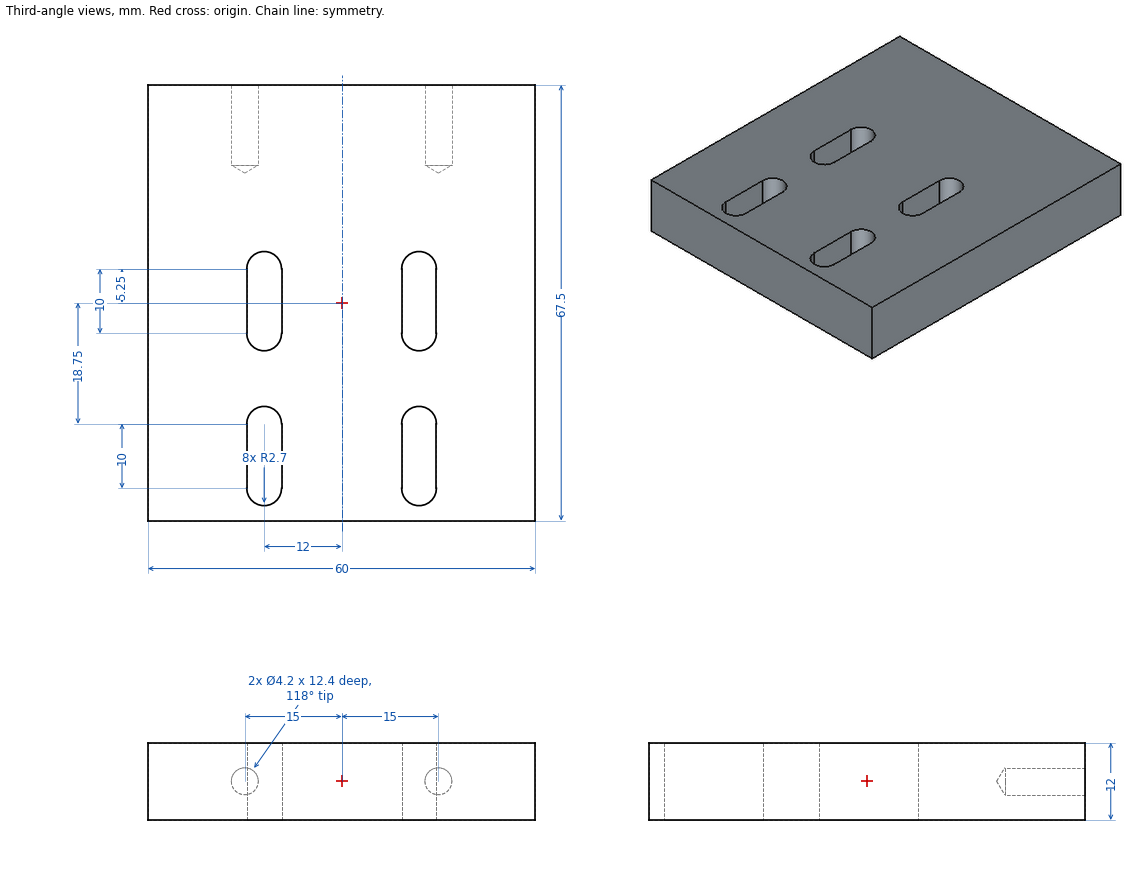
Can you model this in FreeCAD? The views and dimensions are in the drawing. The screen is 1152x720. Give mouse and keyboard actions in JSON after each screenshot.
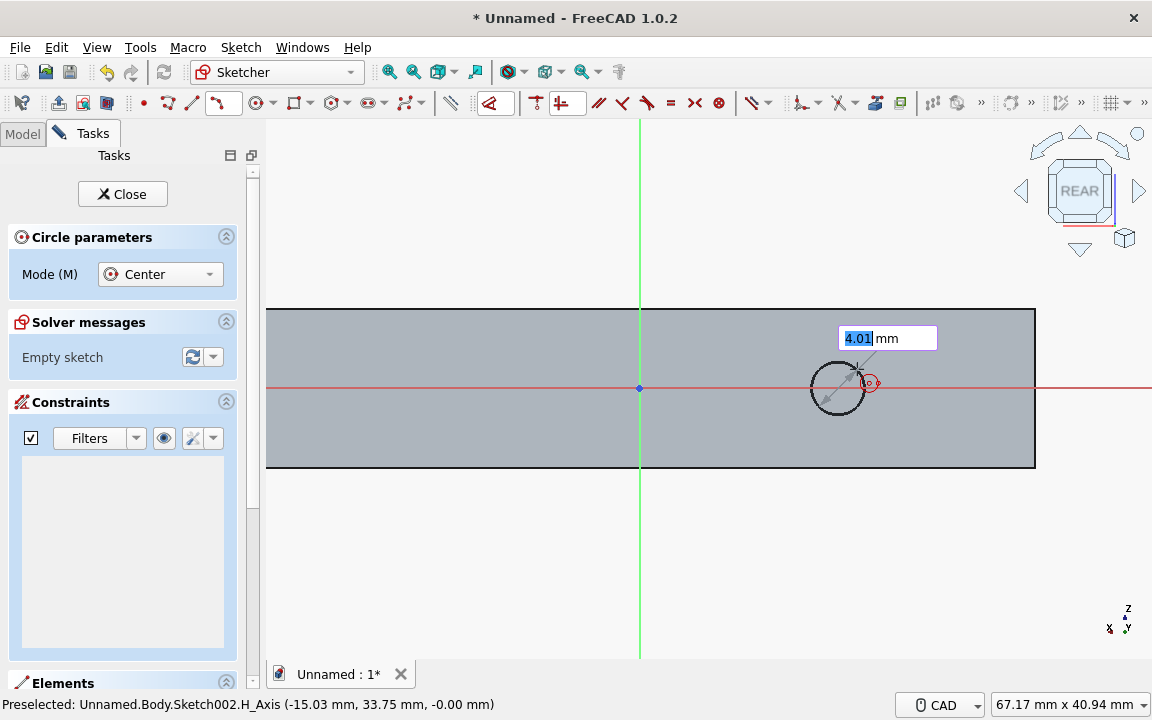
{"action": "type", "text": "4.2"}
{"action": "key", "text": "Return"}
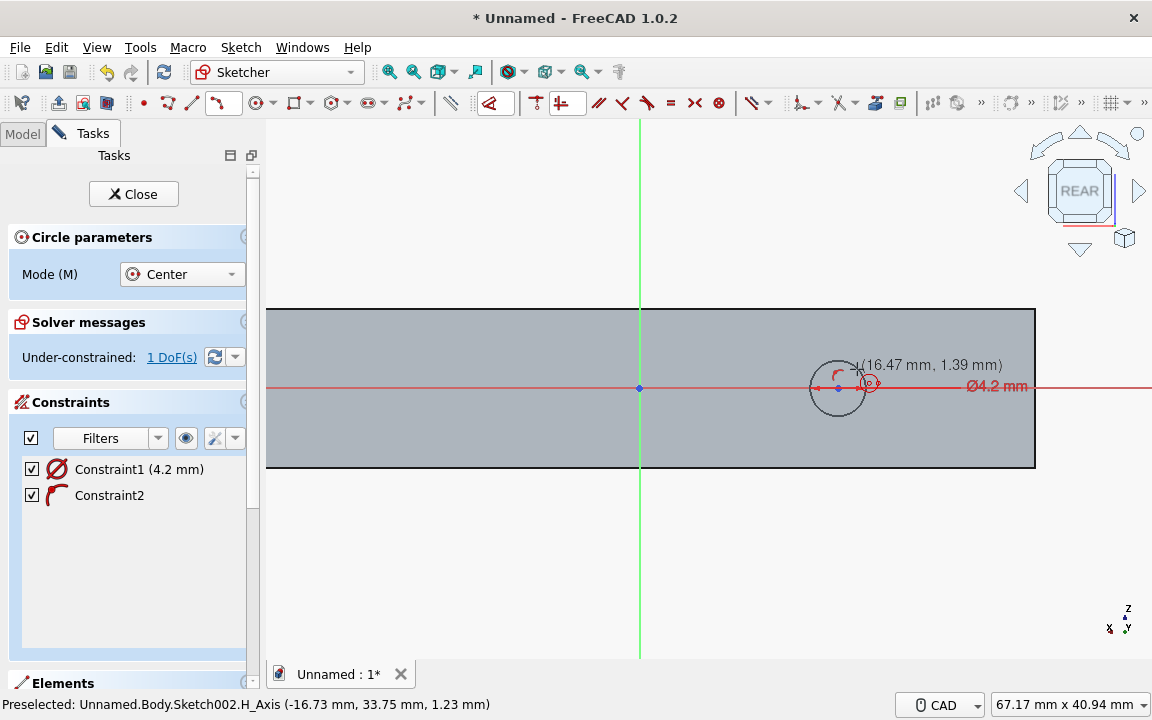
{"action": "left_click", "coordinate": [442, 388]}
{"action": "mouse_move", "coordinate": [461, 369]}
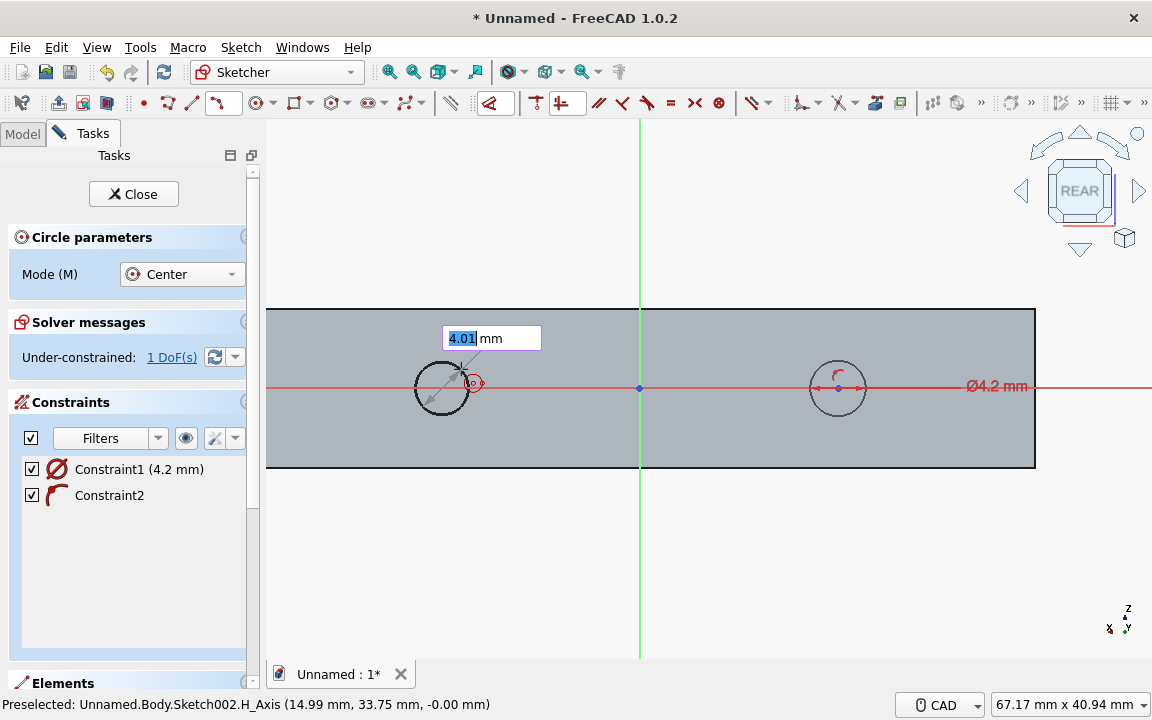
{"action": "type", "text": "4.2"}
{"action": "key", "text": "Return"}
{"action": "key", "text": "Escape"}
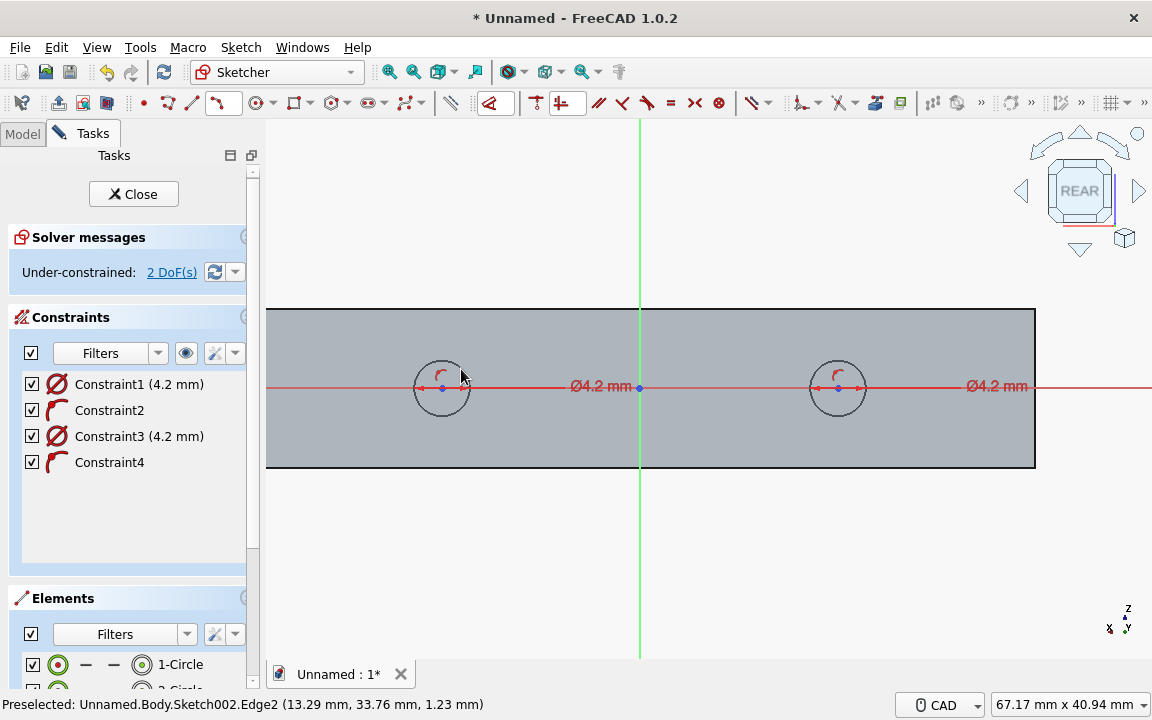
{"action": "left_click", "coordinate": [838, 388]}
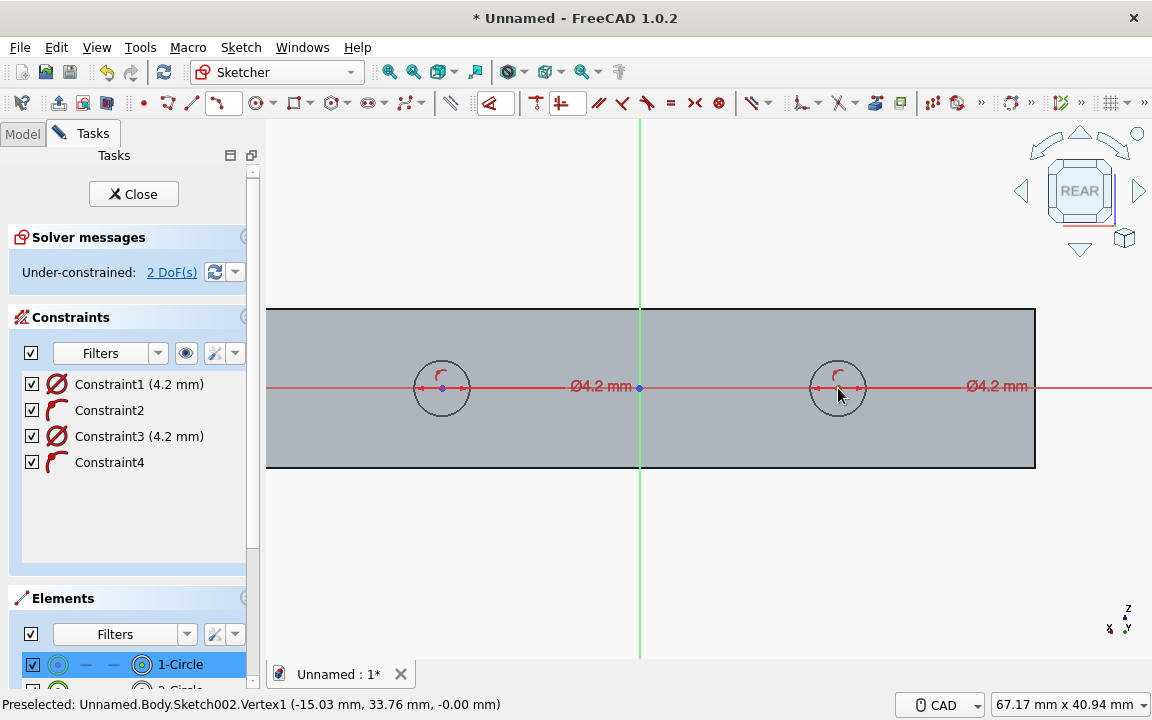
{"action": "left_click", "coordinate": [508, 104]}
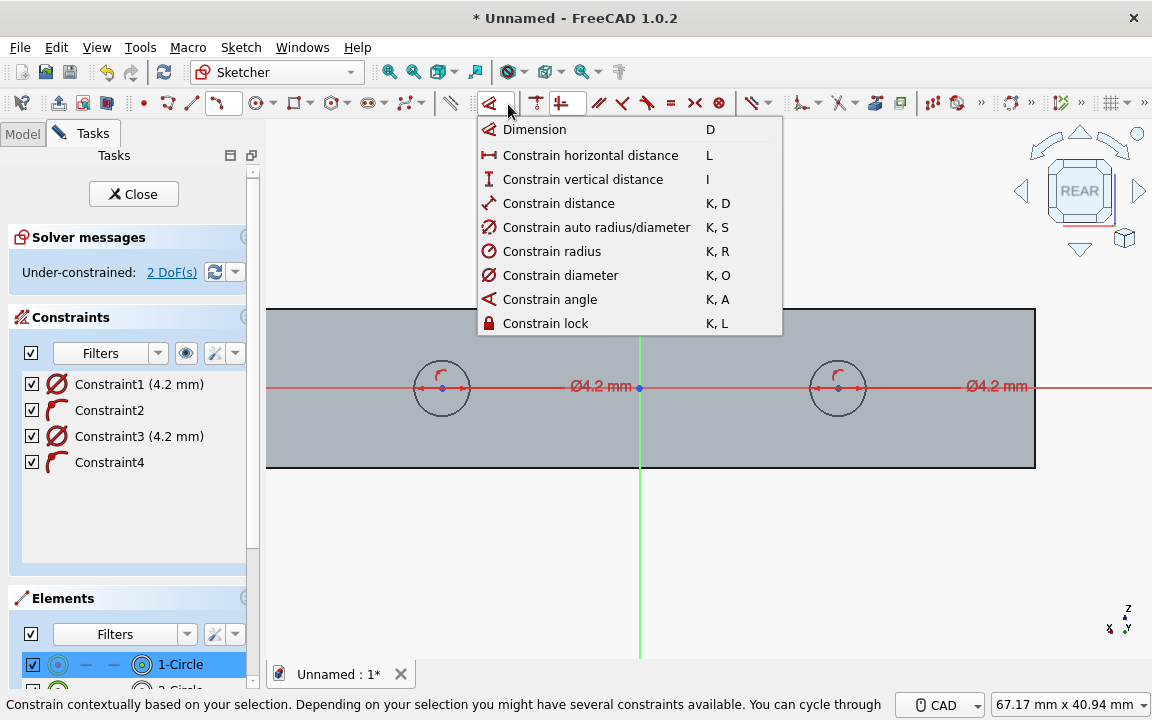
{"action": "left_click", "coordinate": [630, 155]}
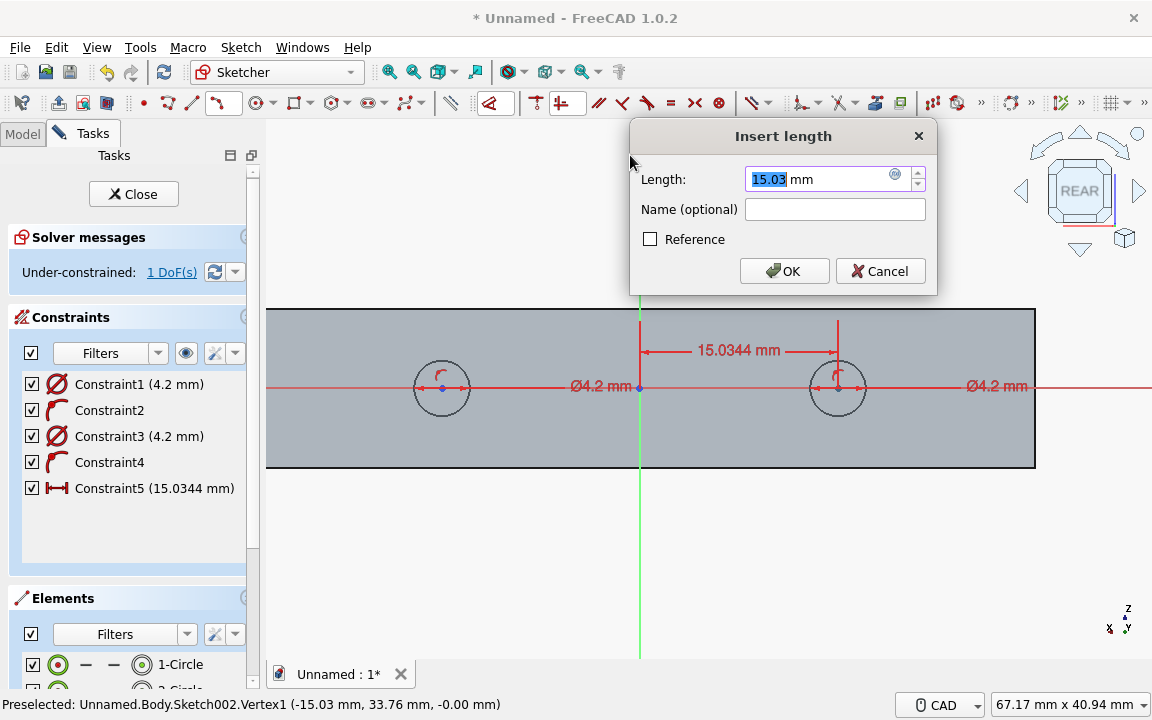
{"action": "type", "text": "15"}
{"action": "key", "text": "Return"}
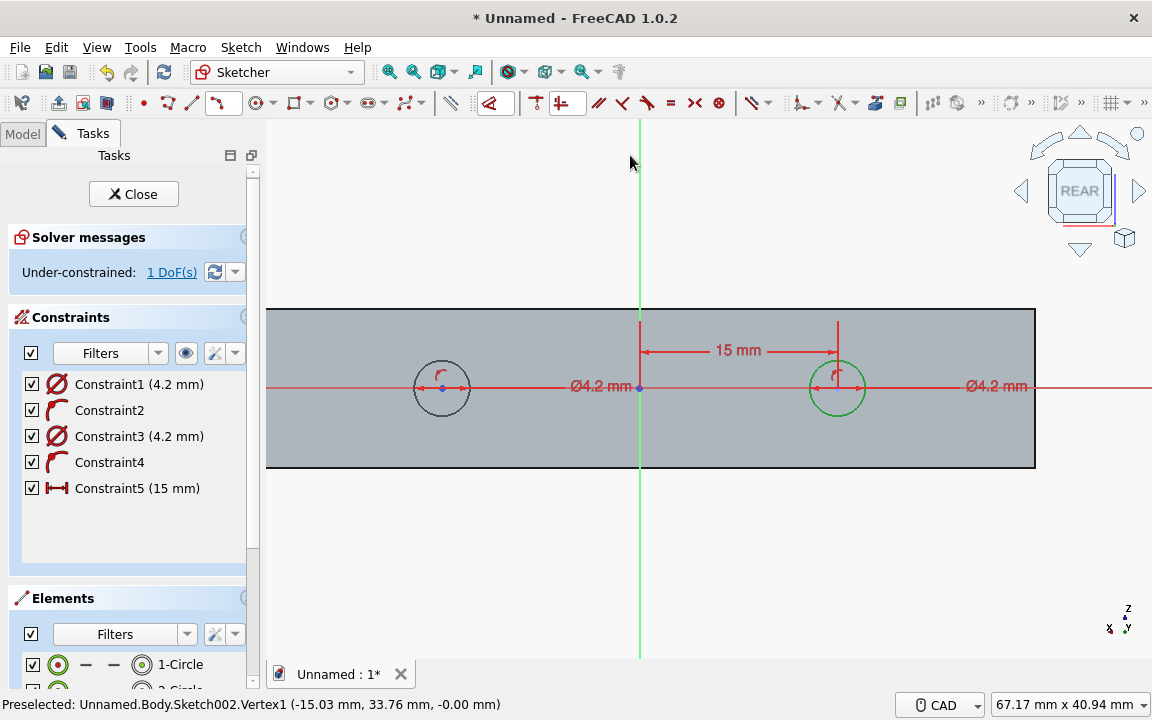
{"action": "left_click", "coordinate": [442, 388]}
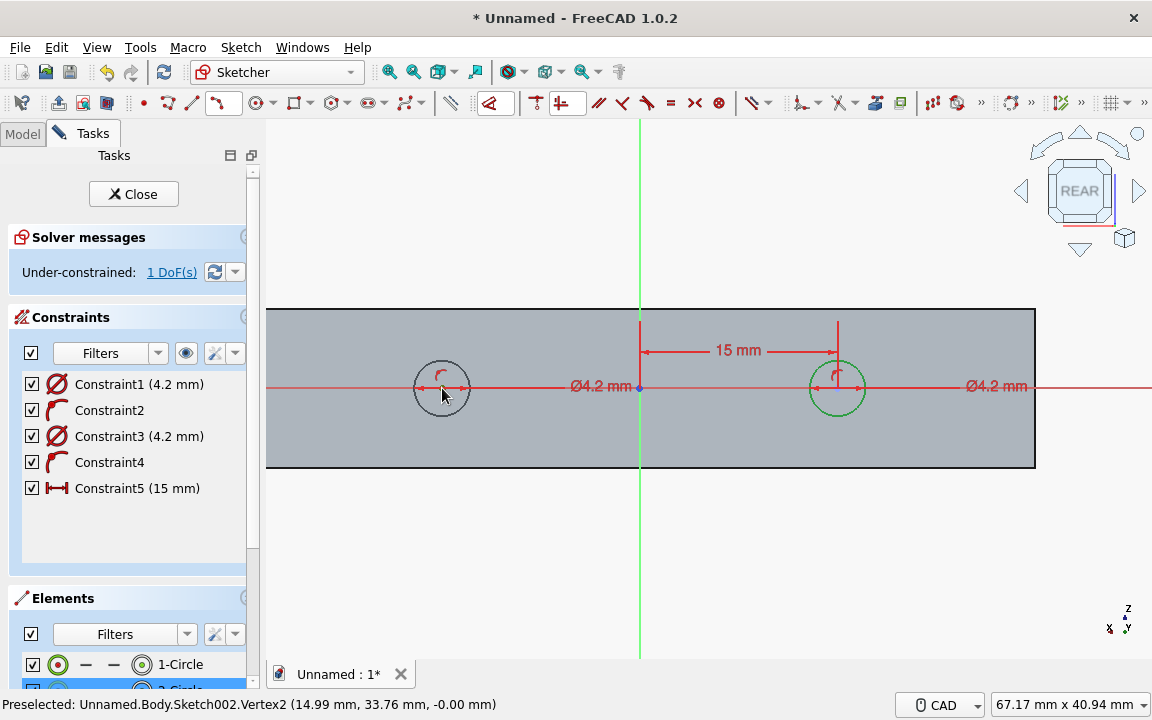
{"action": "key", "text": "l"}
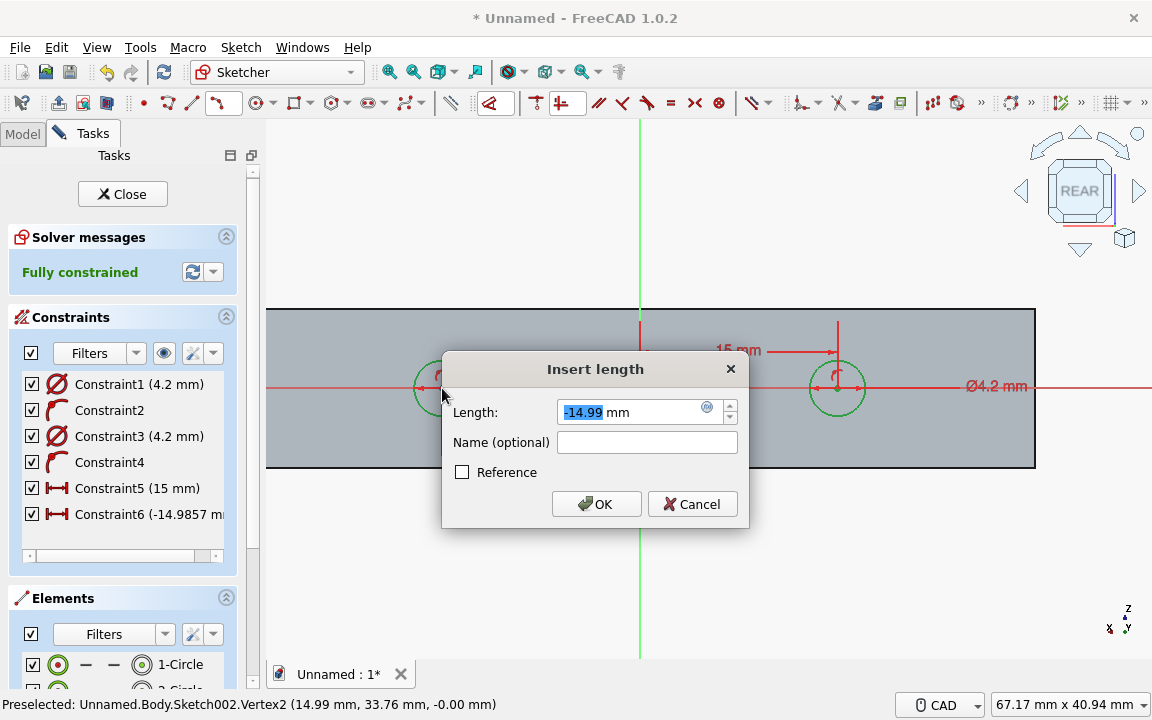
{"action": "type", "text": "-15"}
{"action": "key", "text": "Return"}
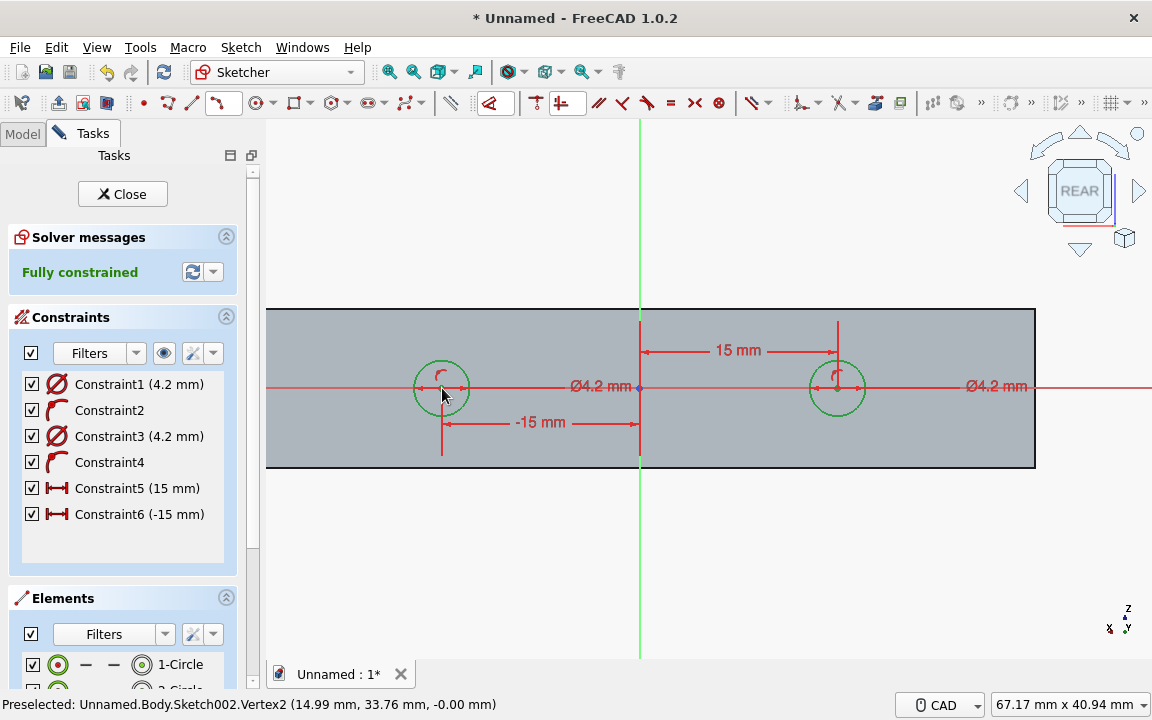
{"action": "left_click", "coordinate": [123, 194]}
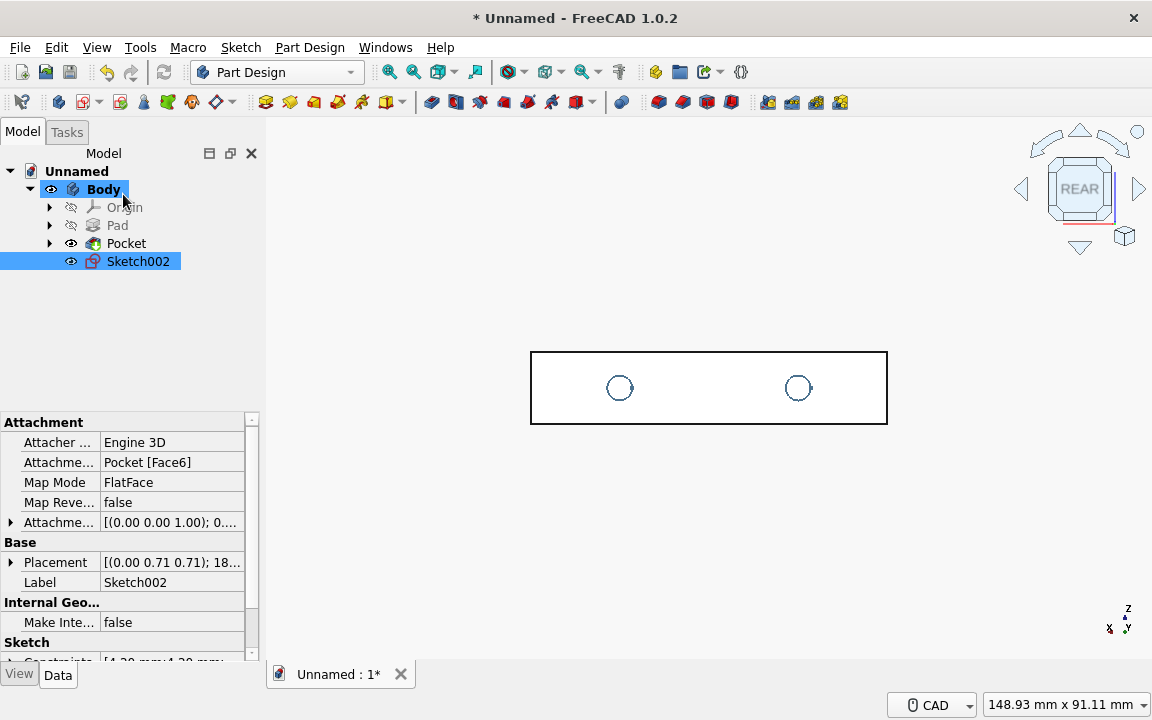
{"action": "left_click", "coordinate": [456, 102]}